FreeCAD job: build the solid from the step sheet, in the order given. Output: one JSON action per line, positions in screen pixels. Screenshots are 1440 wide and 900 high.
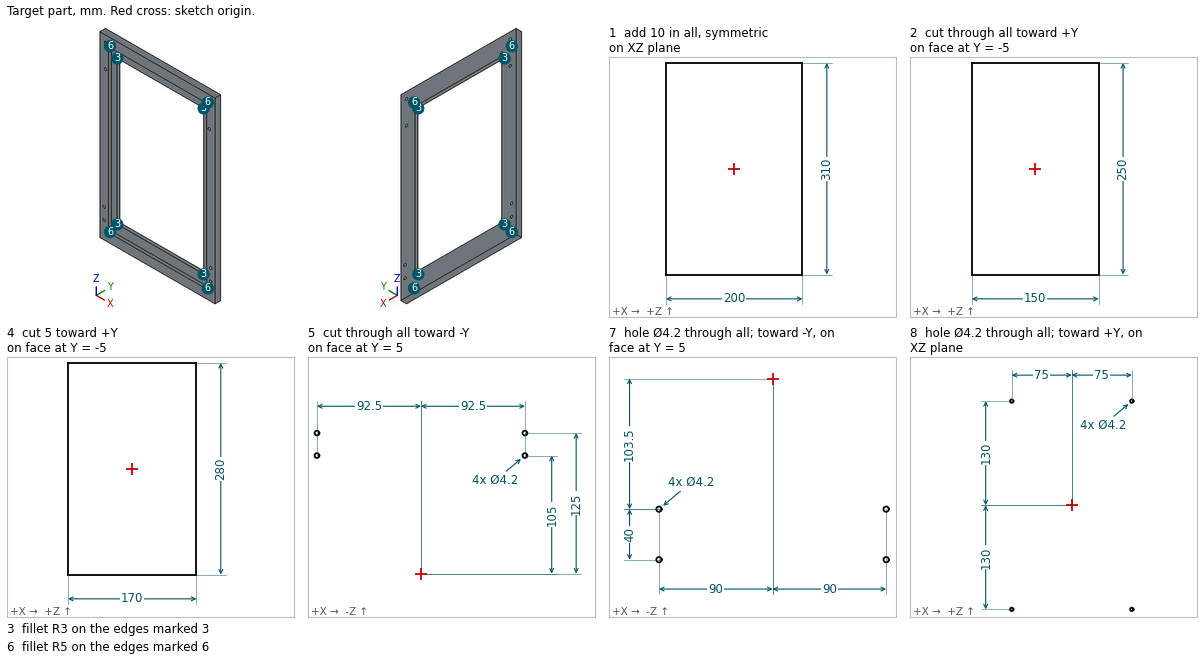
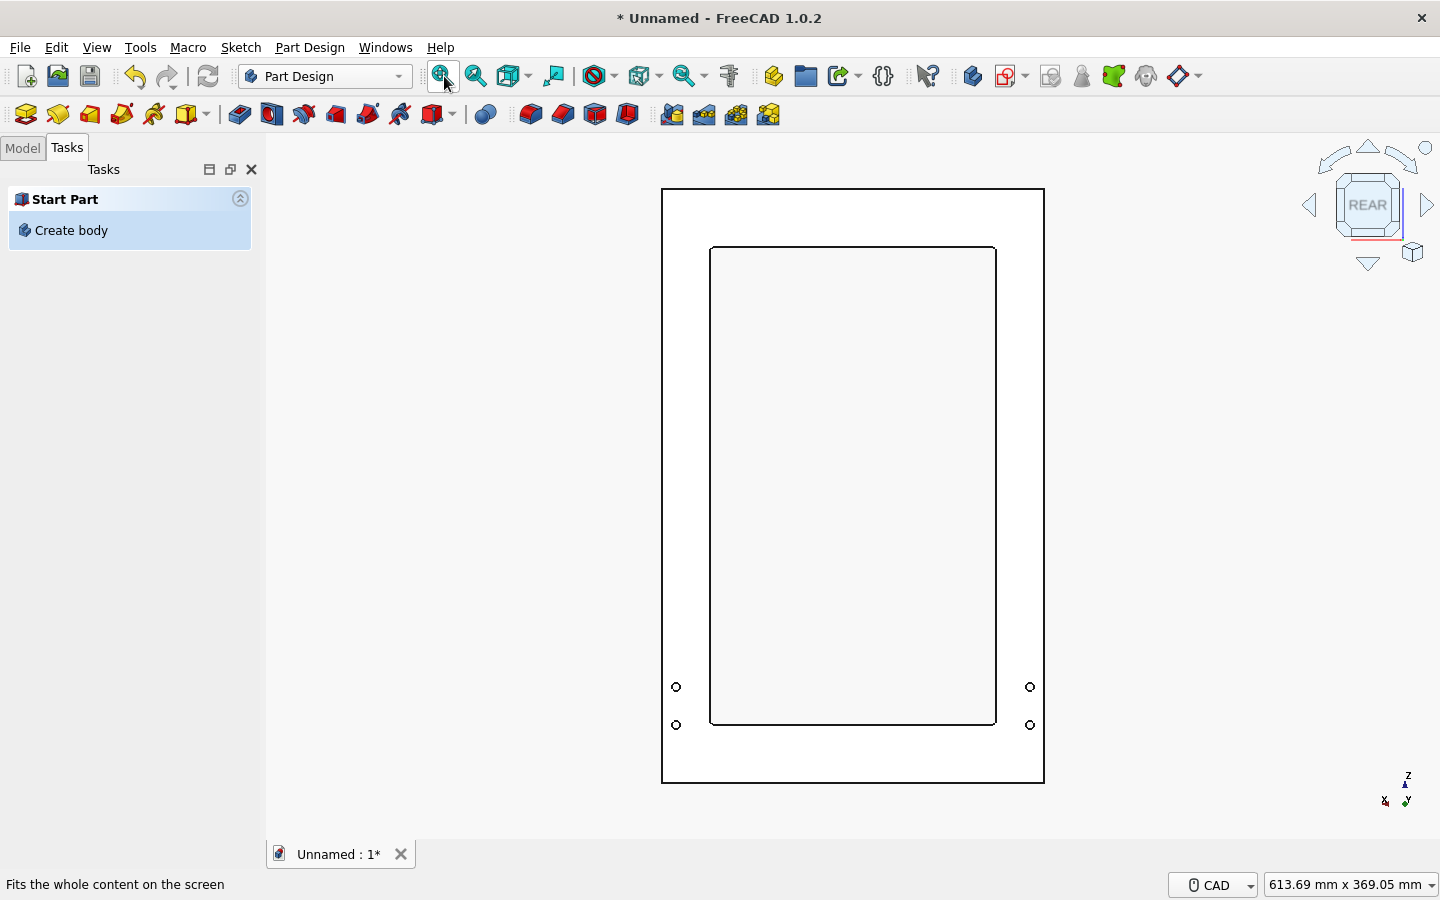
{"action": "key", "text": "6"}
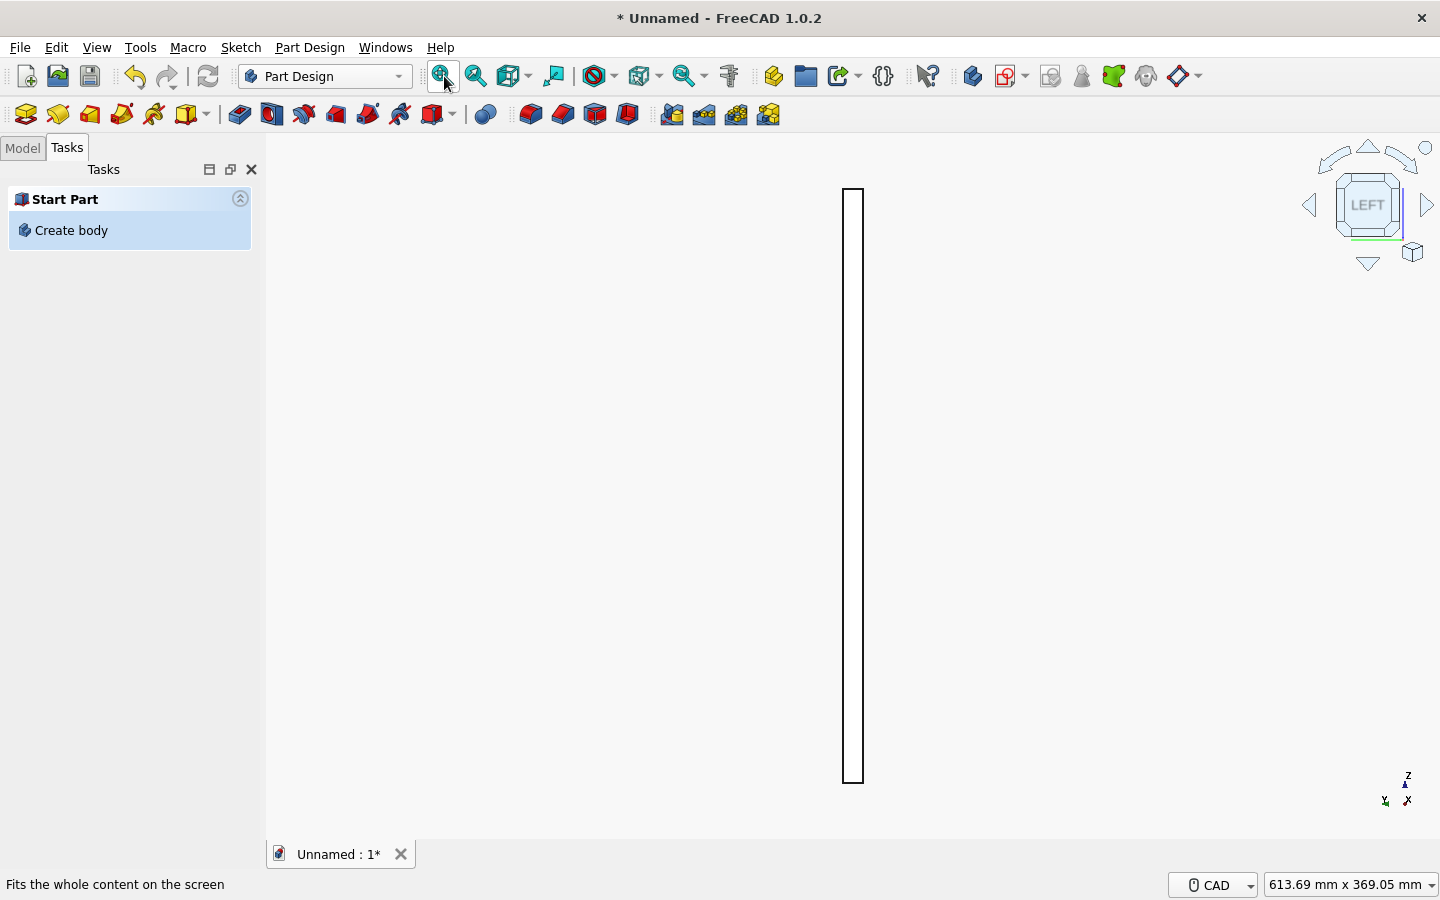
{"action": "scroll", "coordinate": [858, 217], "scroll_direction": "up", "scroll_amount": 8}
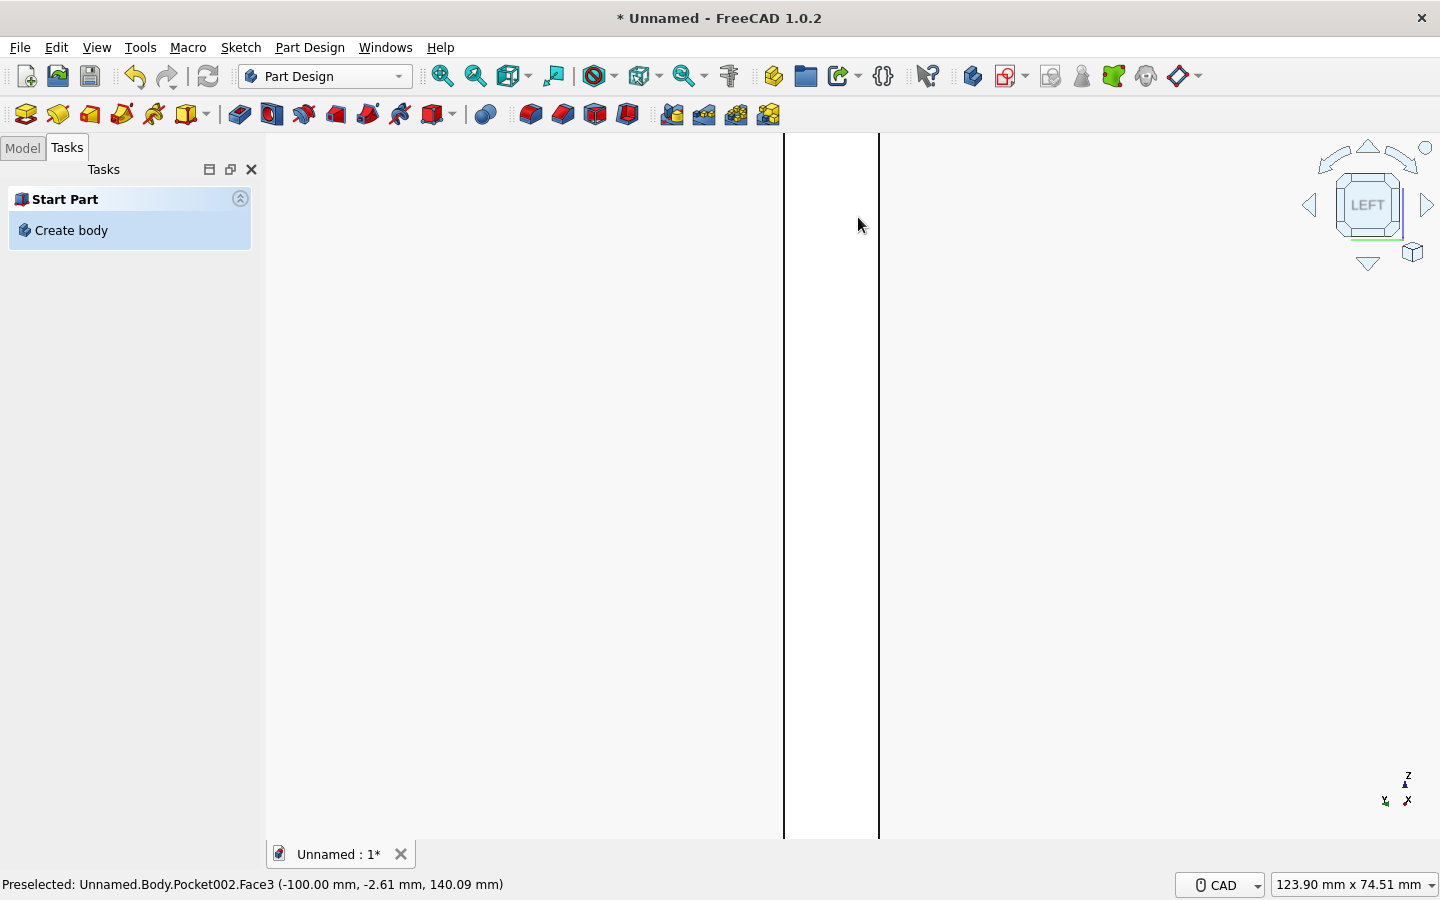
{"action": "key", "text": "v f"}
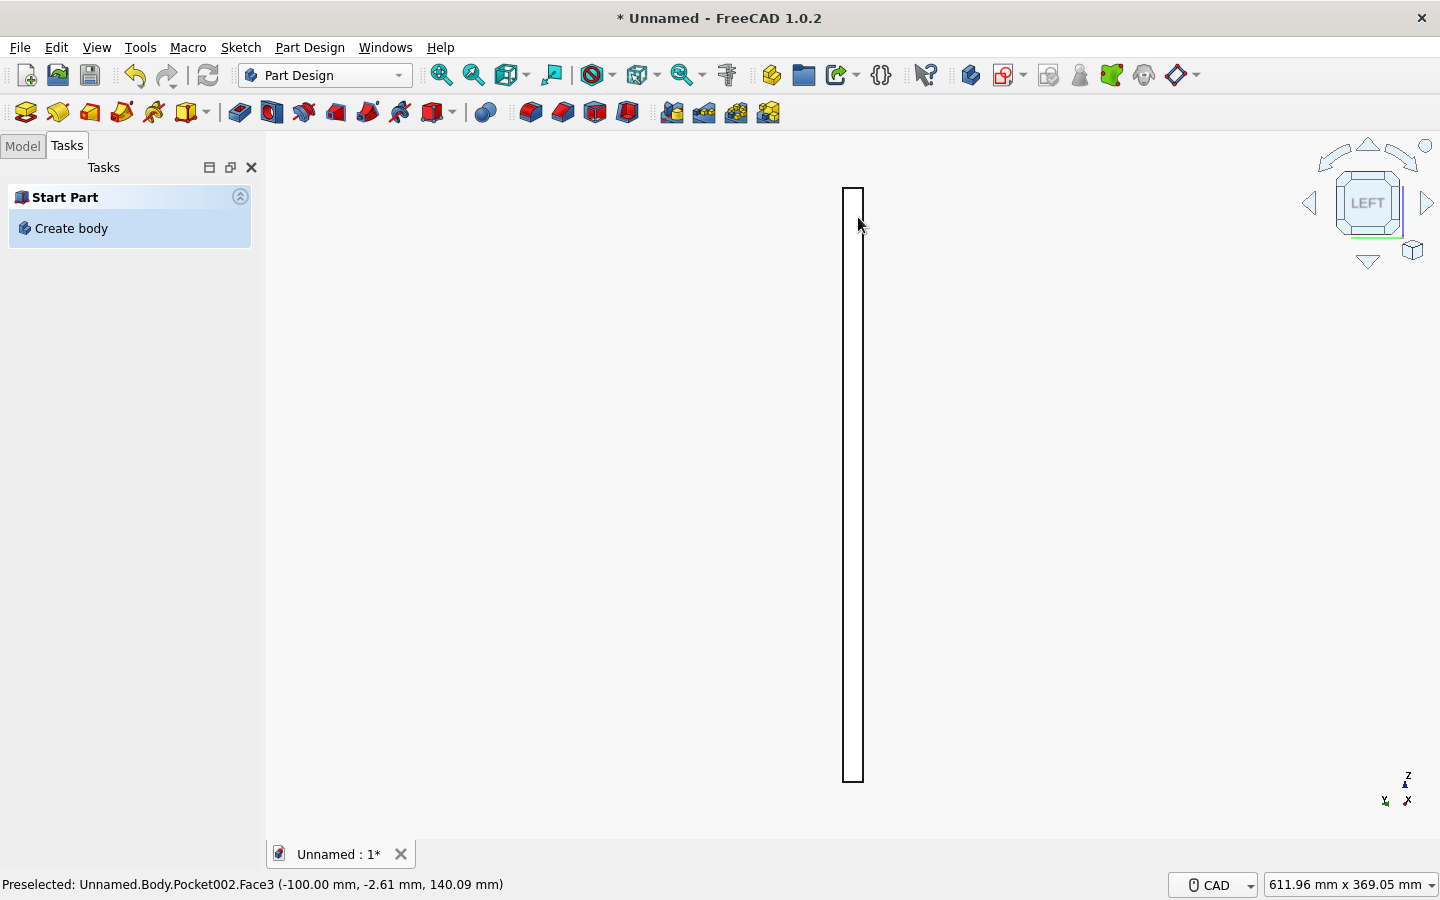
{"action": "key", "text": "v 3"}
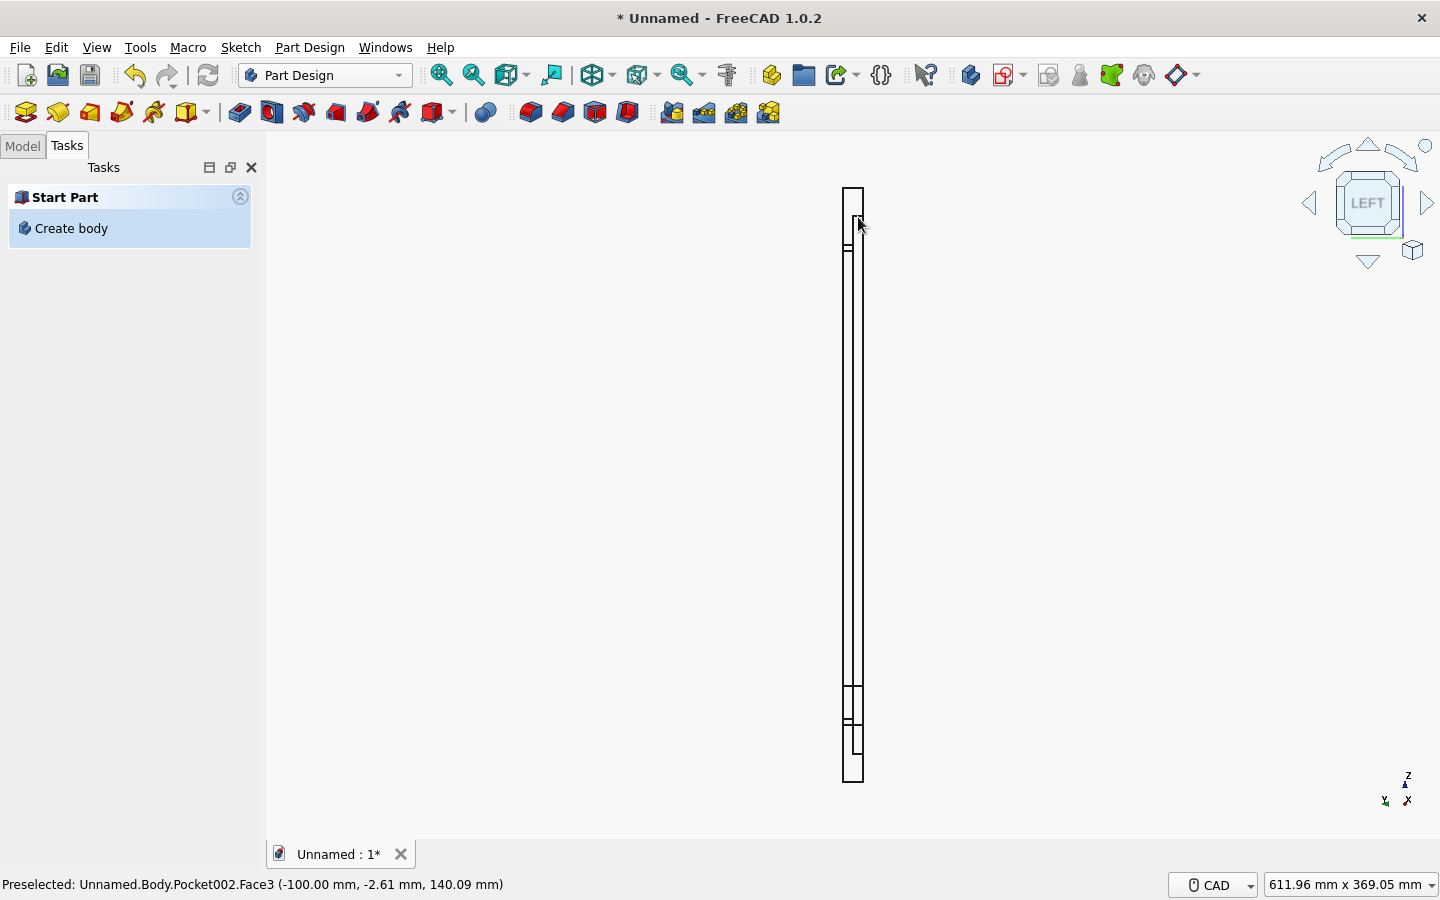
{"action": "key", "text": "0"}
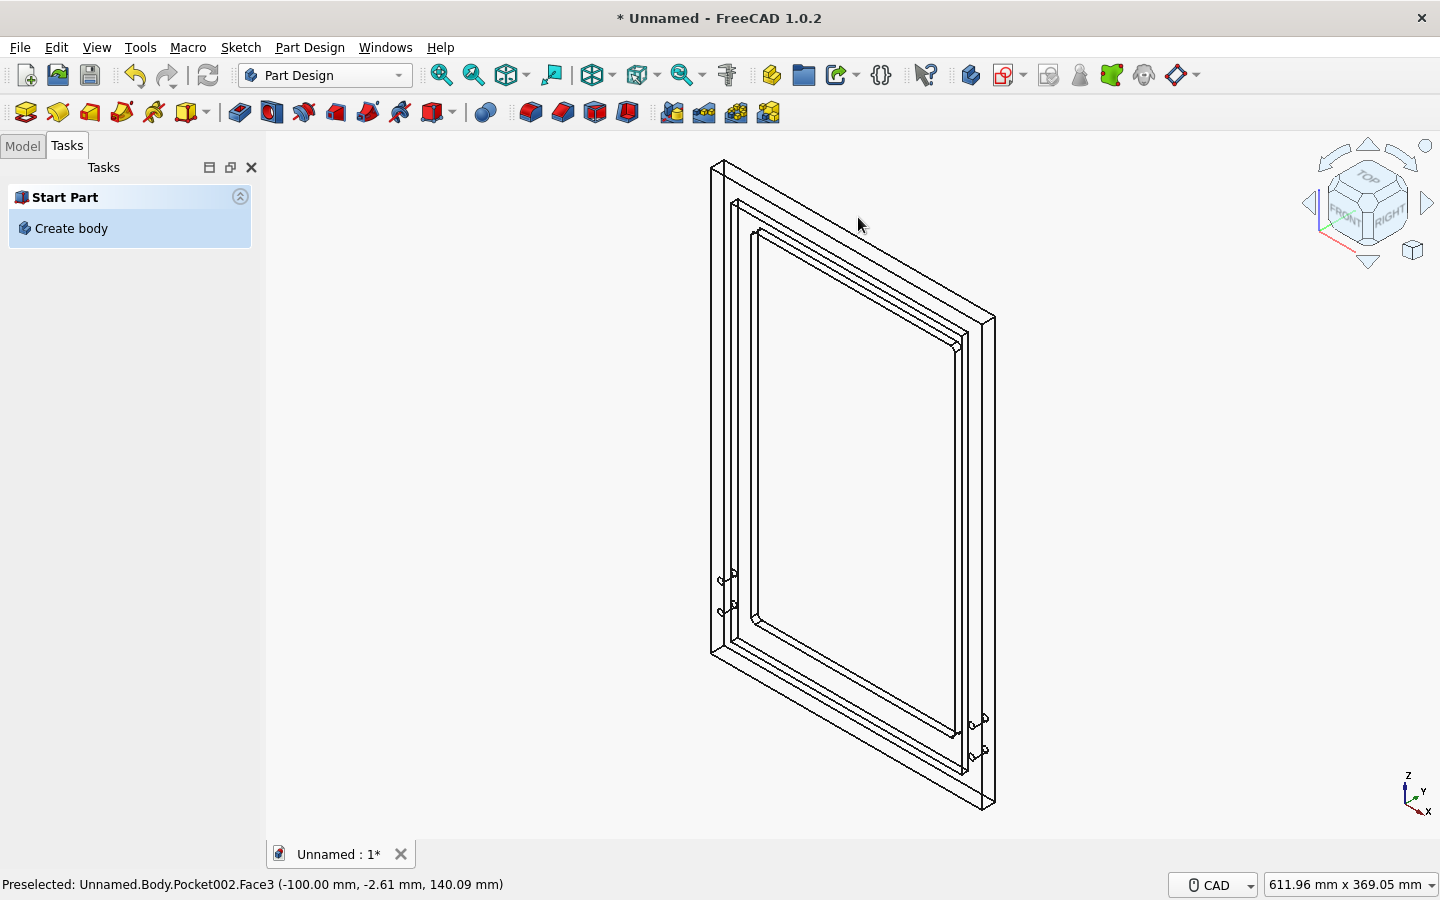
{"action": "scroll", "coordinate": [965, 333], "scroll_direction": "up", "scroll_amount": 8}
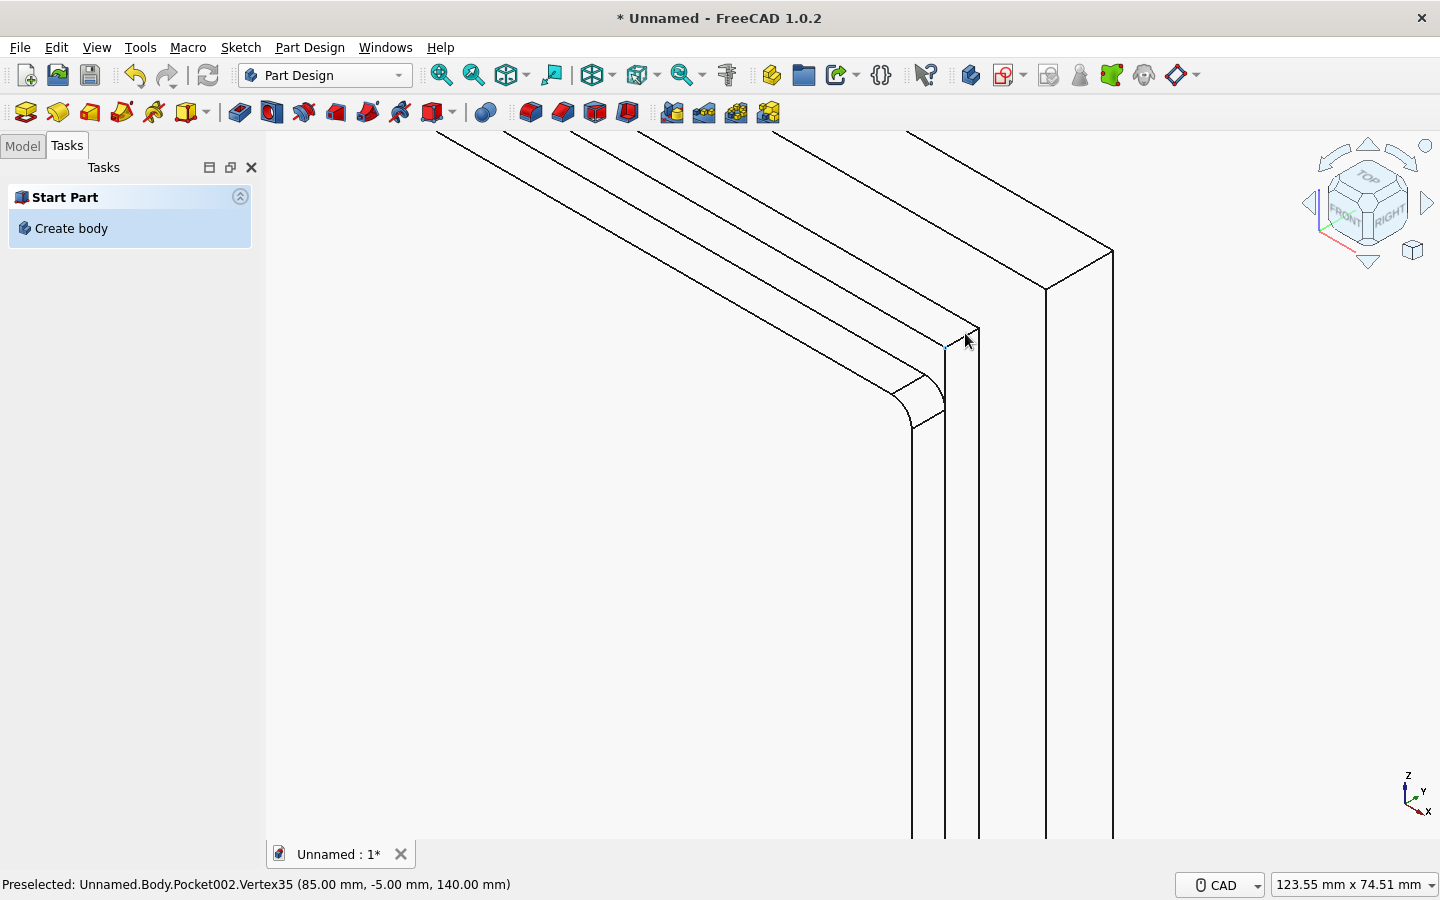
{"action": "left_click", "coordinate": [962, 337]}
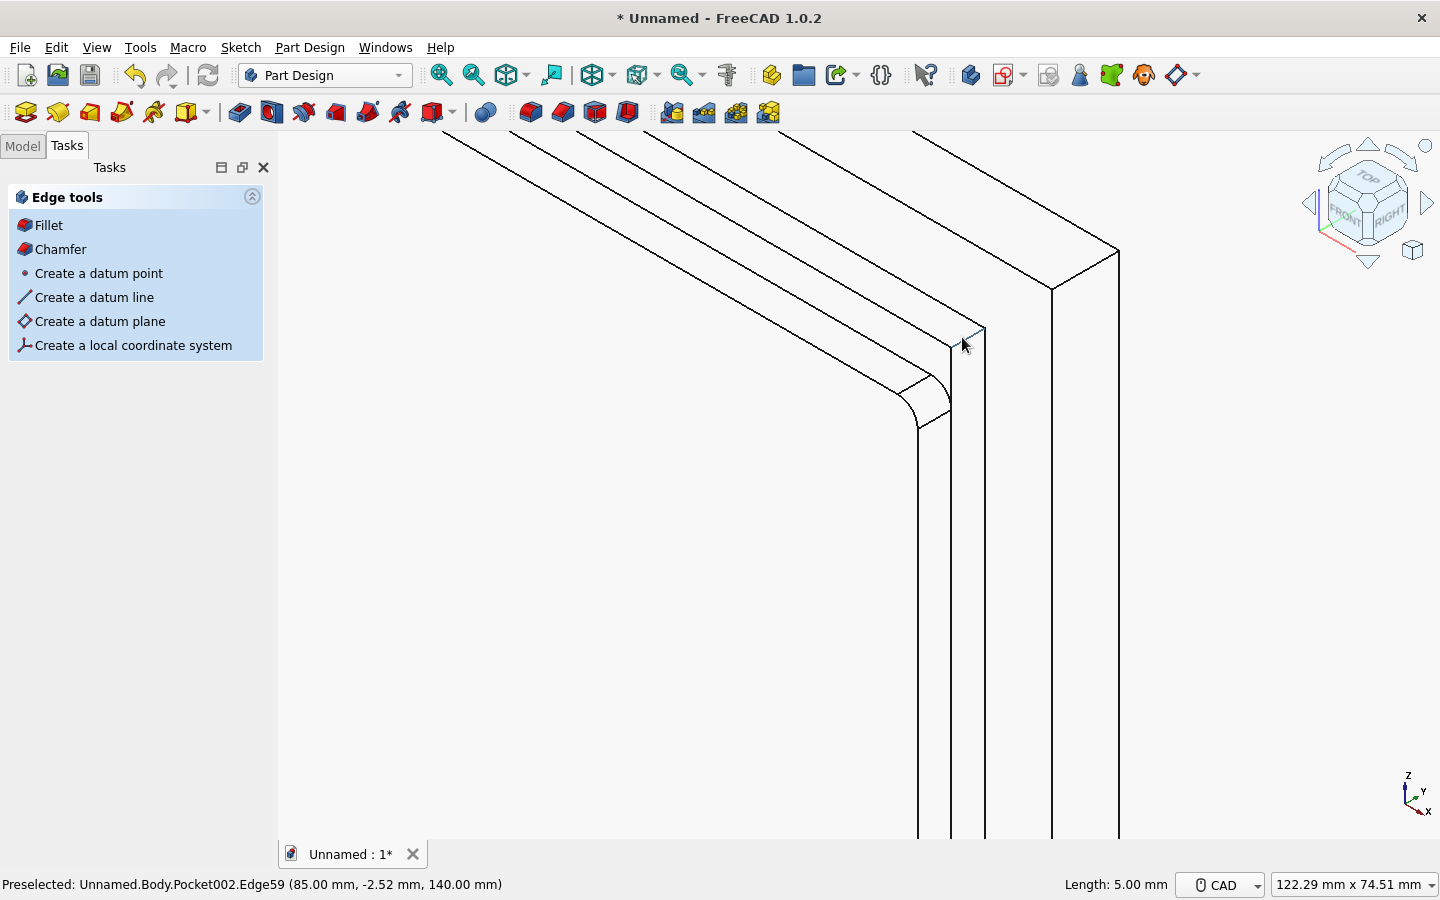
{"action": "left_click", "coordinate": [442, 76]}